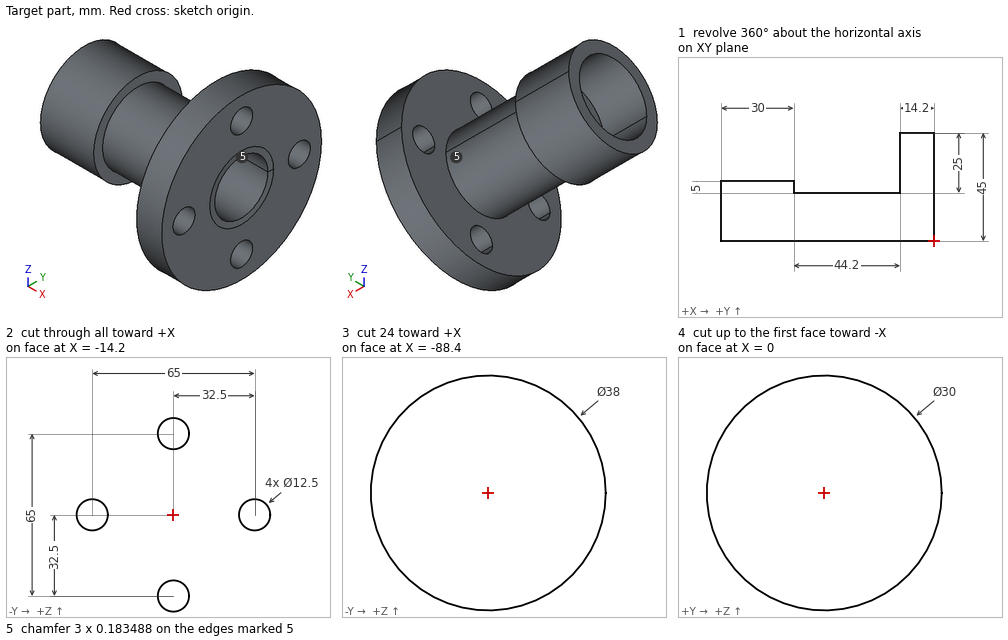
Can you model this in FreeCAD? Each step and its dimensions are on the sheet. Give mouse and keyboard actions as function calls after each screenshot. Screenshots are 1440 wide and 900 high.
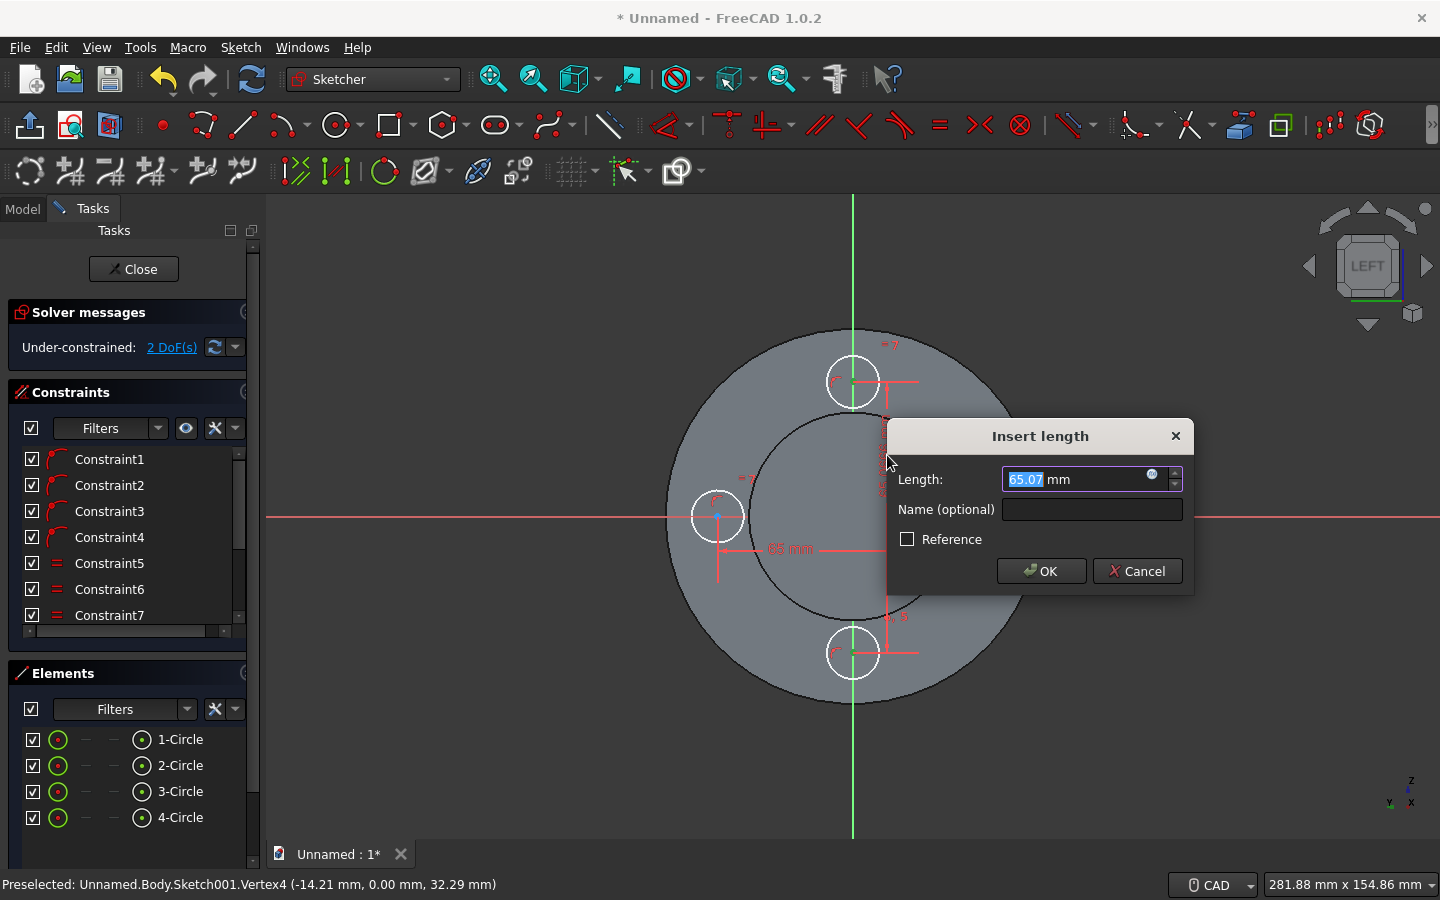
text(65)
key(Return)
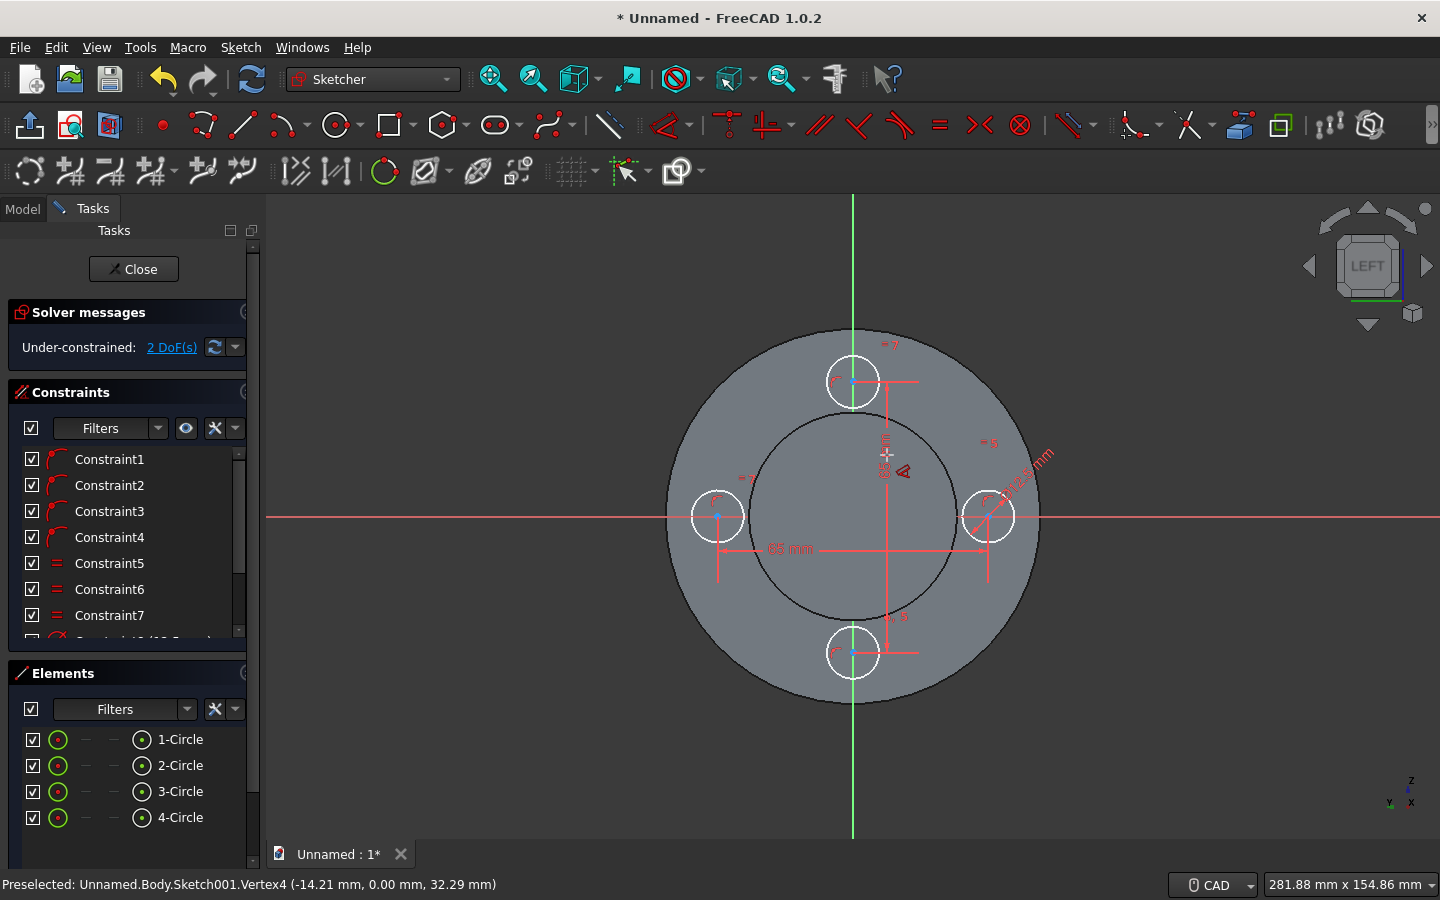
click(988, 516)
click(921, 550)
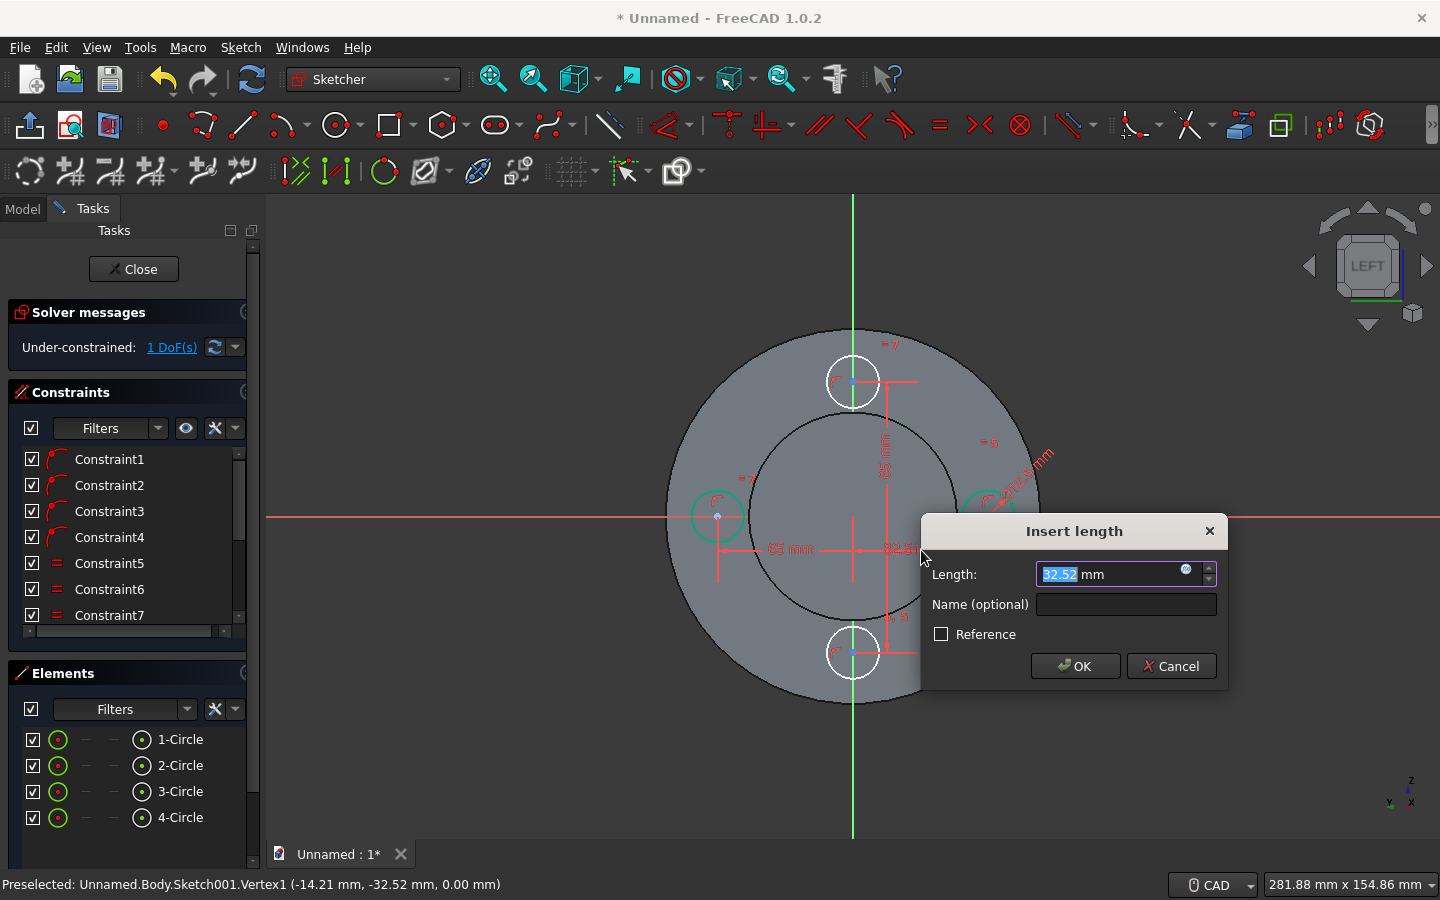
text(32.5)
key(Return)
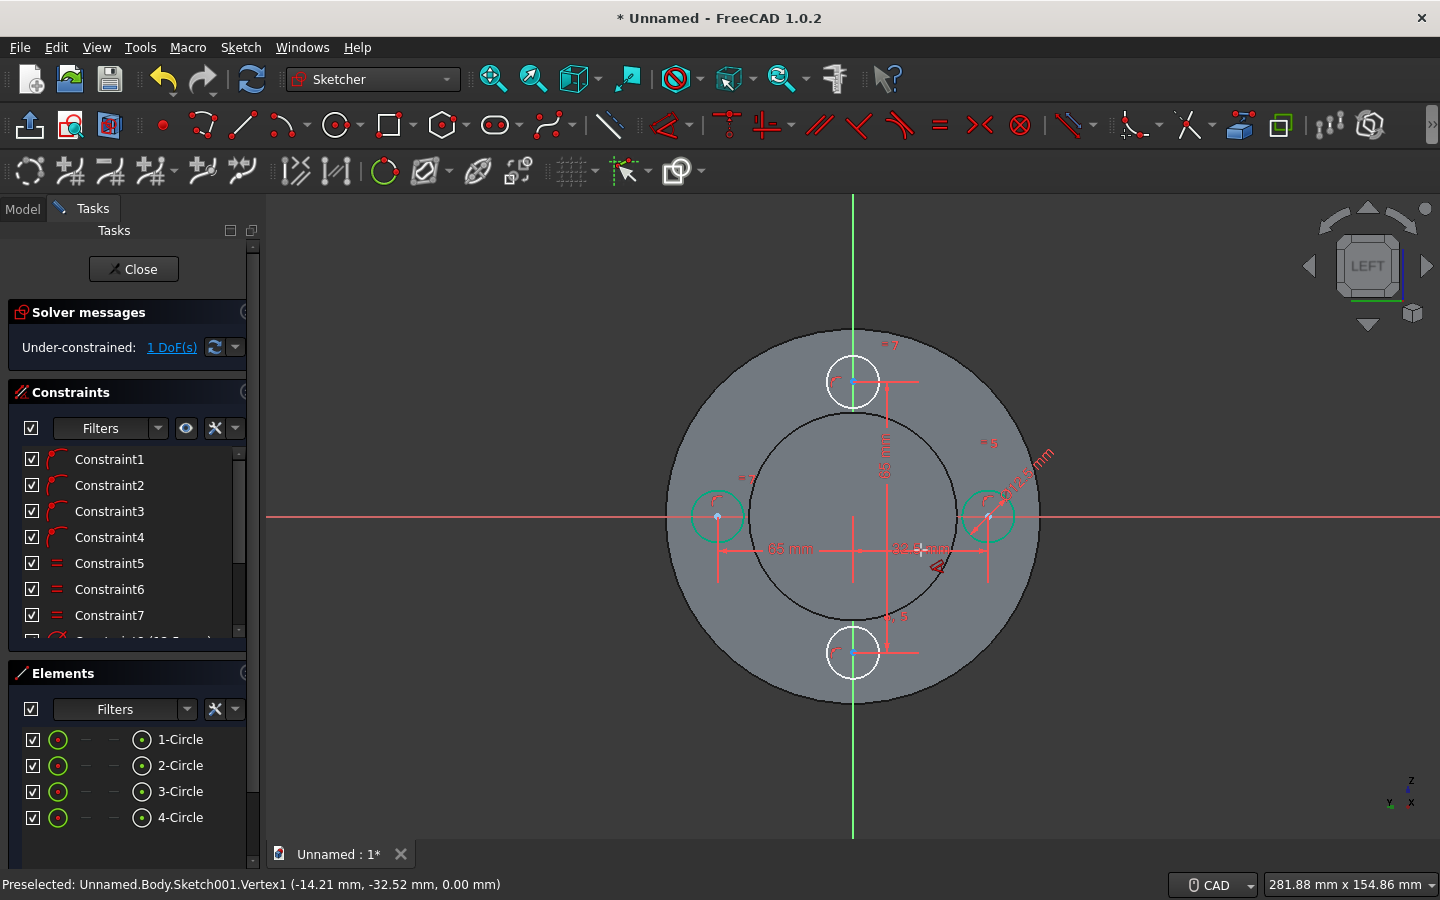
click(853, 653)
click(887, 585)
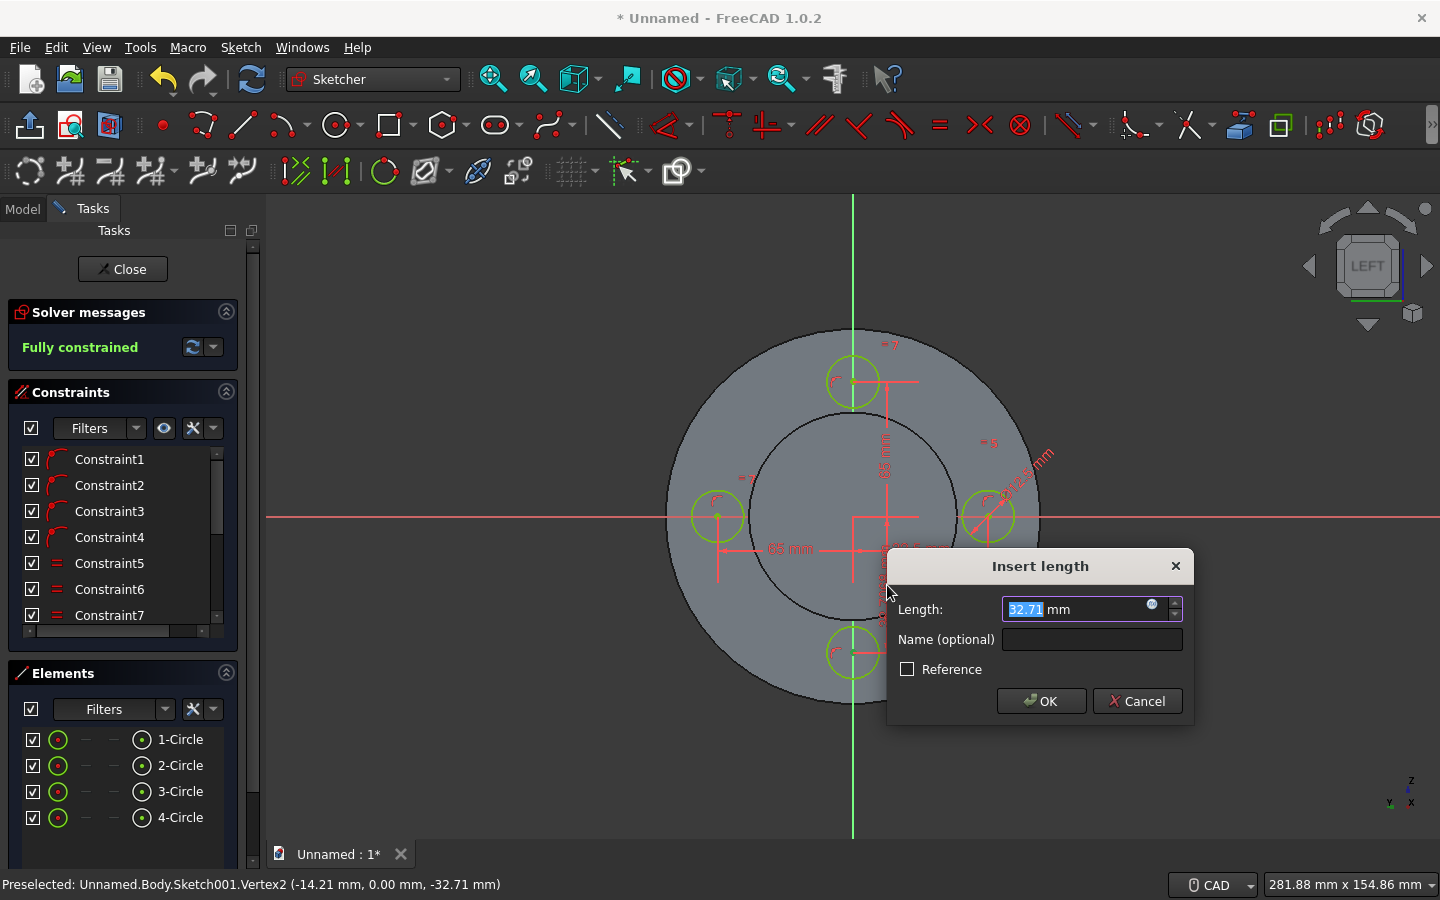
text(32.5)
key(Return)
key(Escape)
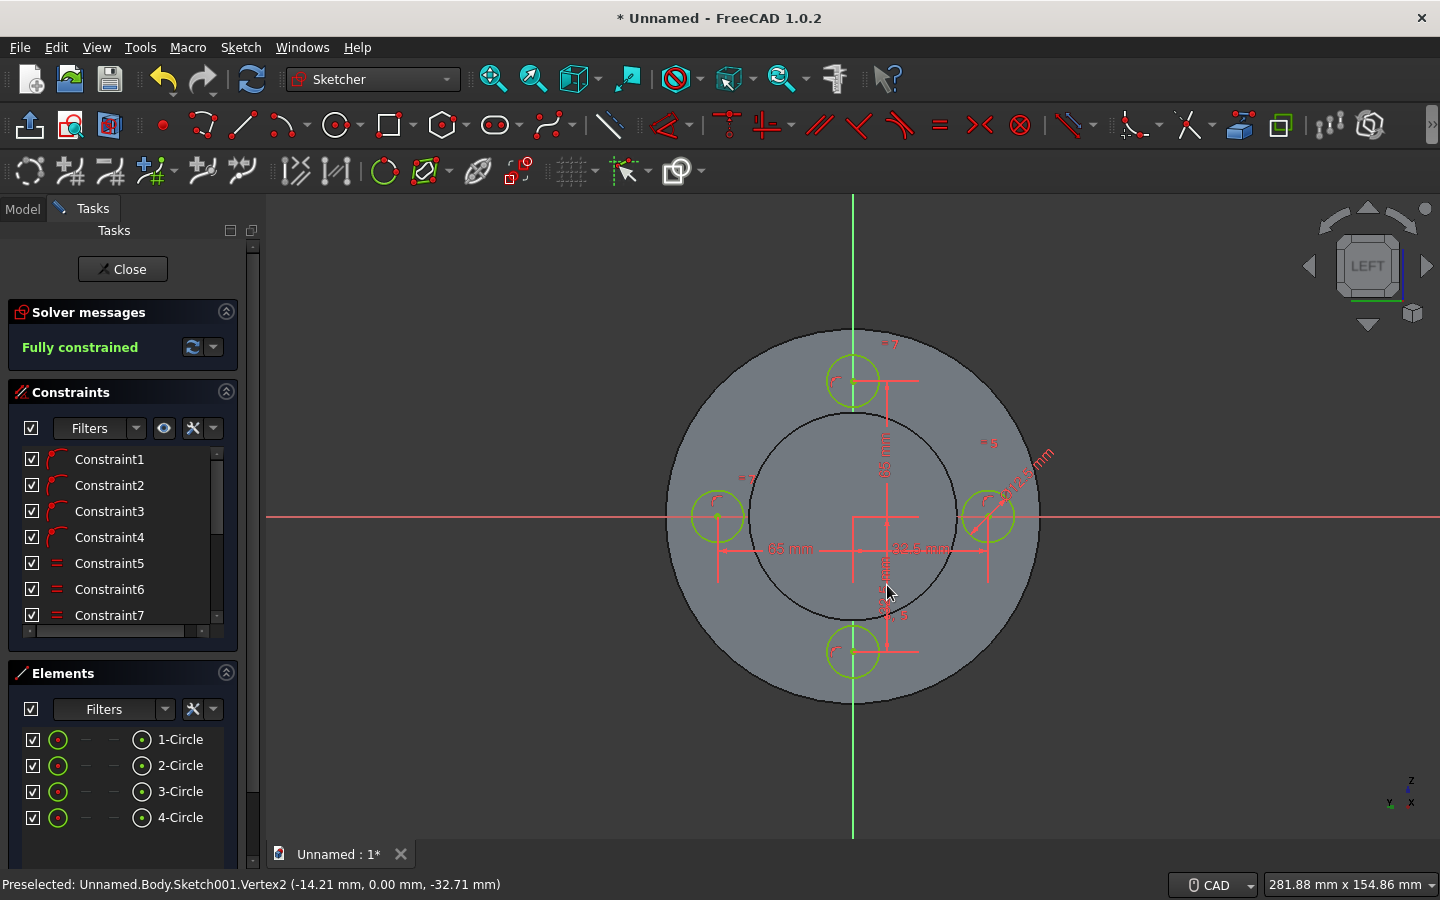
click(123, 269)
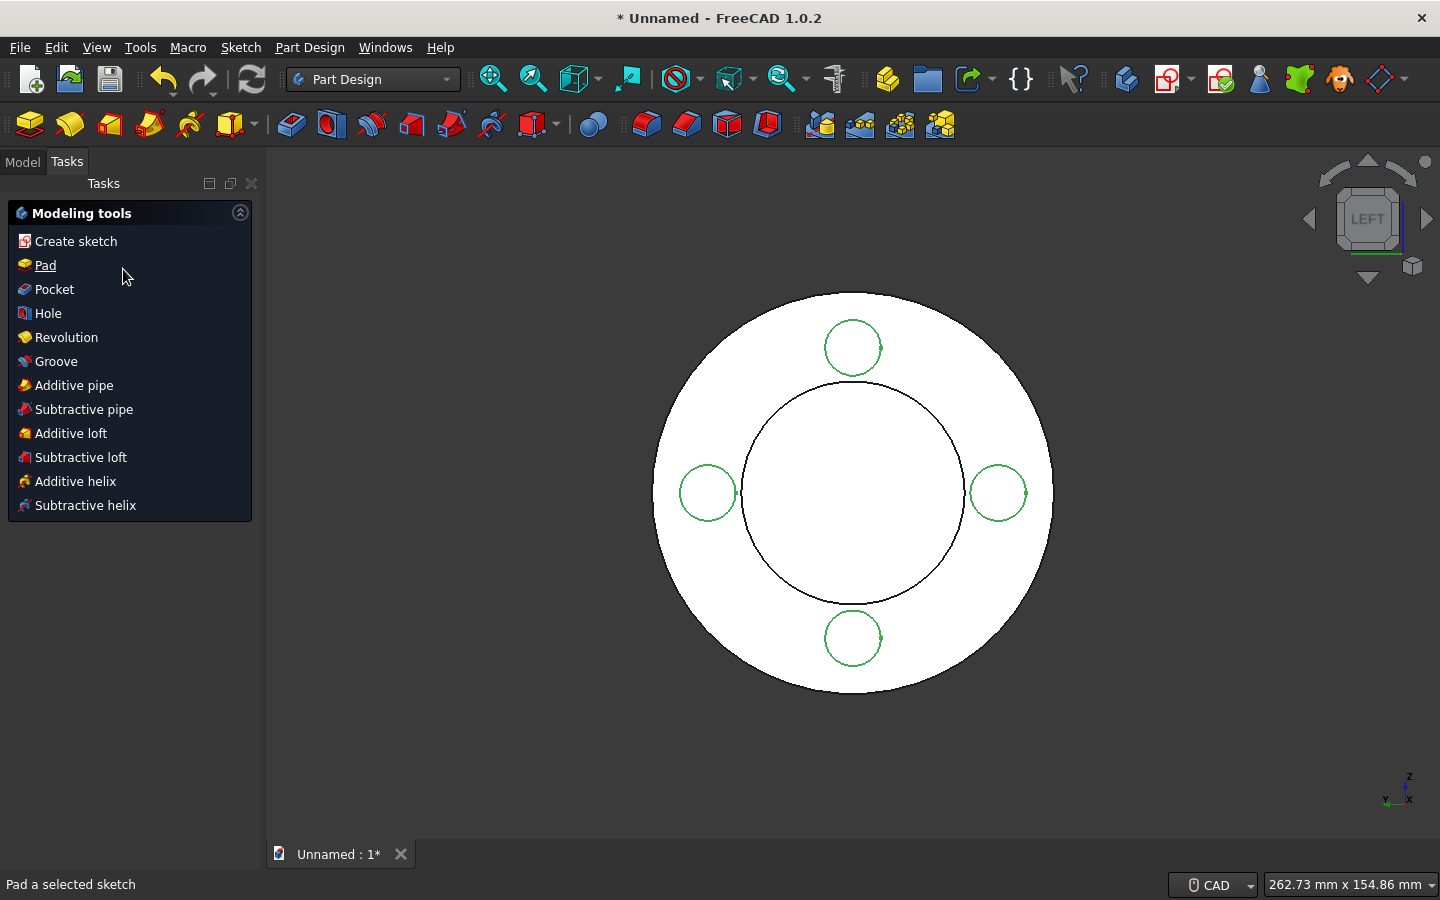
click(292, 124)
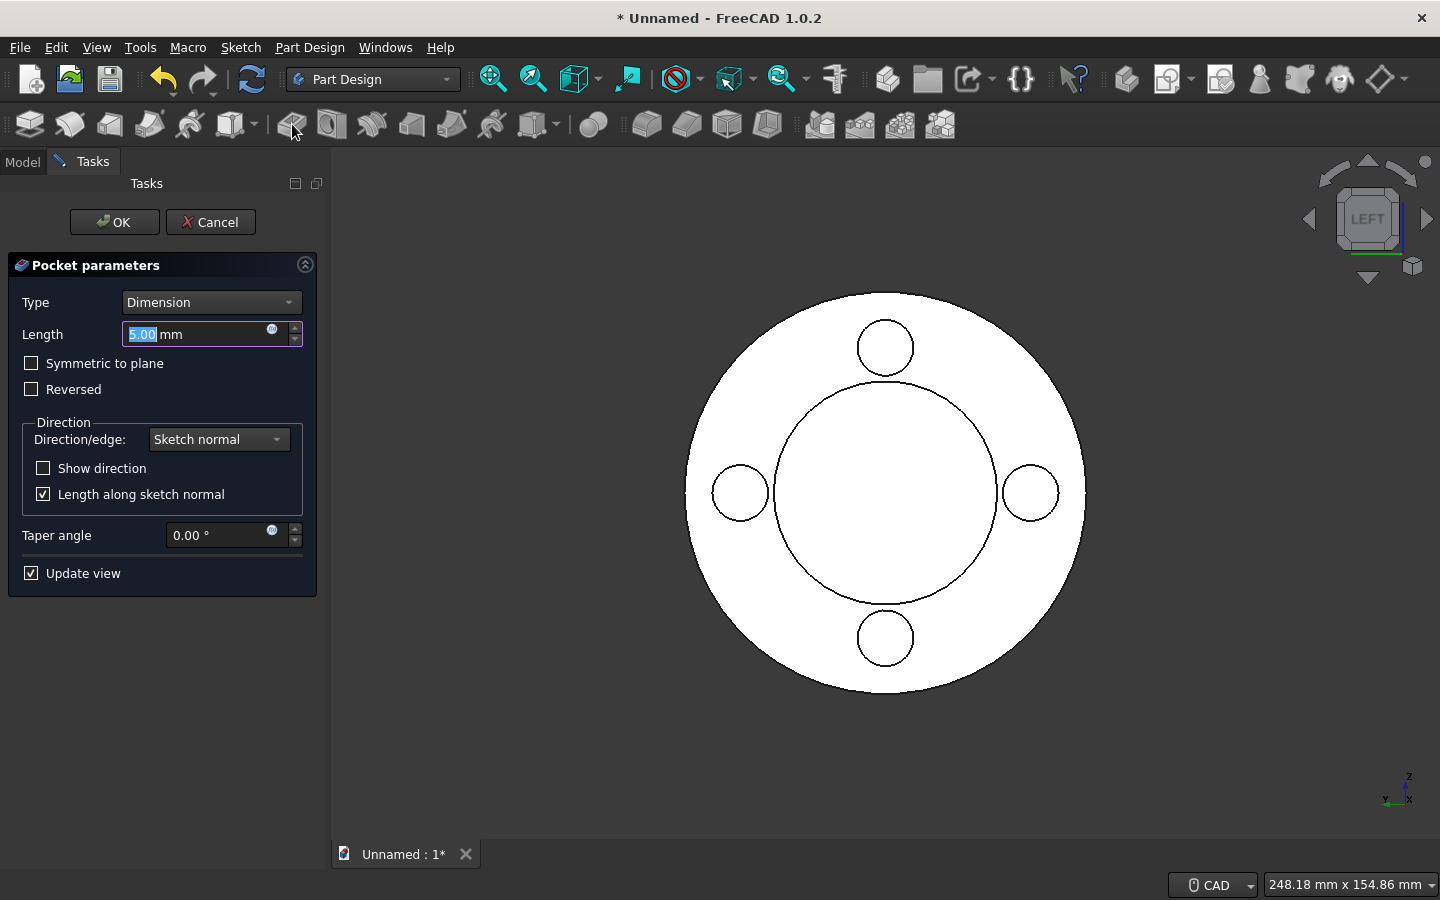
click(212, 302)